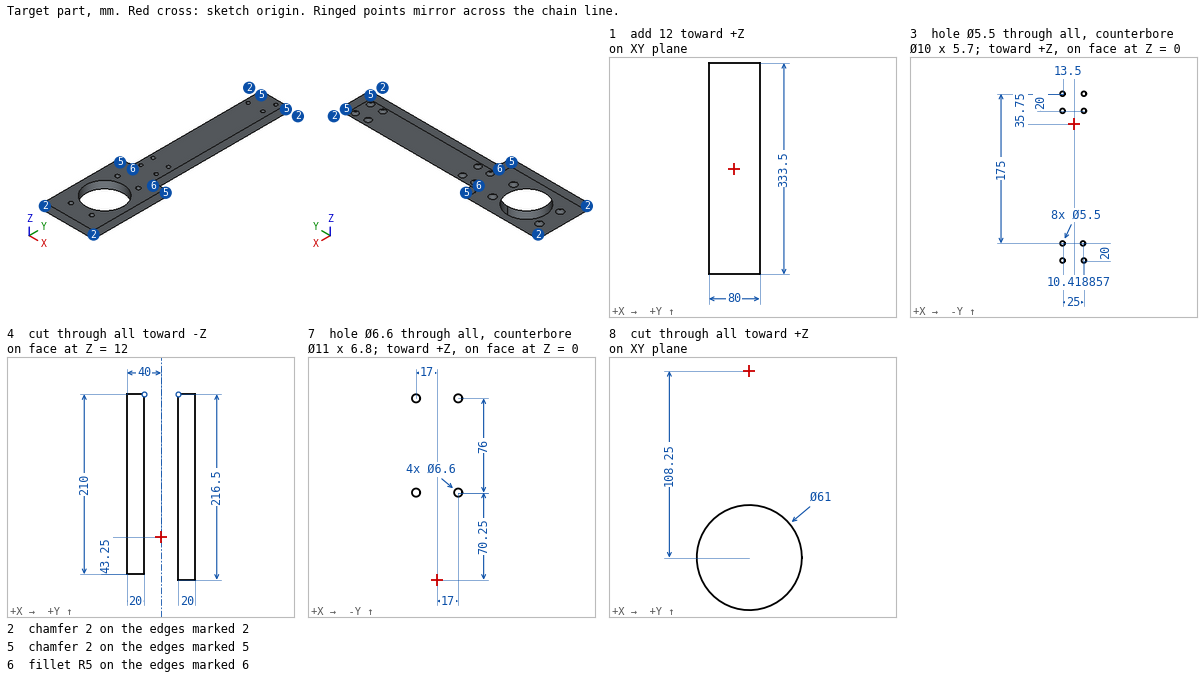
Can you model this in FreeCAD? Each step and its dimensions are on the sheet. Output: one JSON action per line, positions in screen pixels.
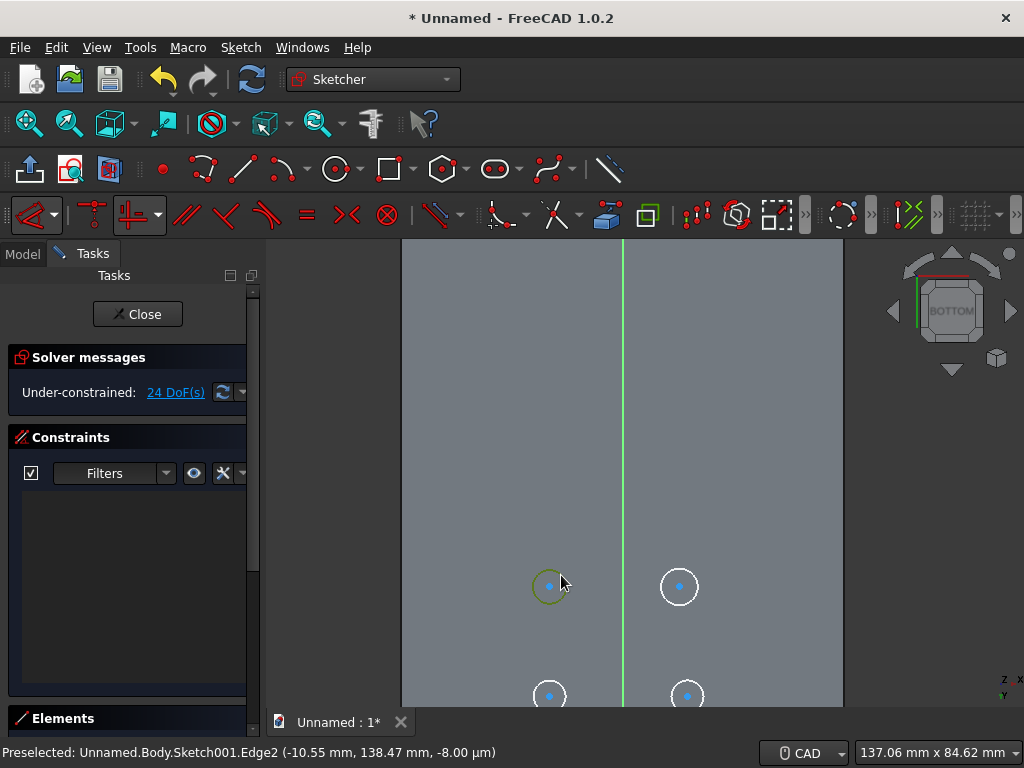
{"action": "scroll", "coordinate": [563, 577], "scroll_direction": "down", "scroll_amount": 7}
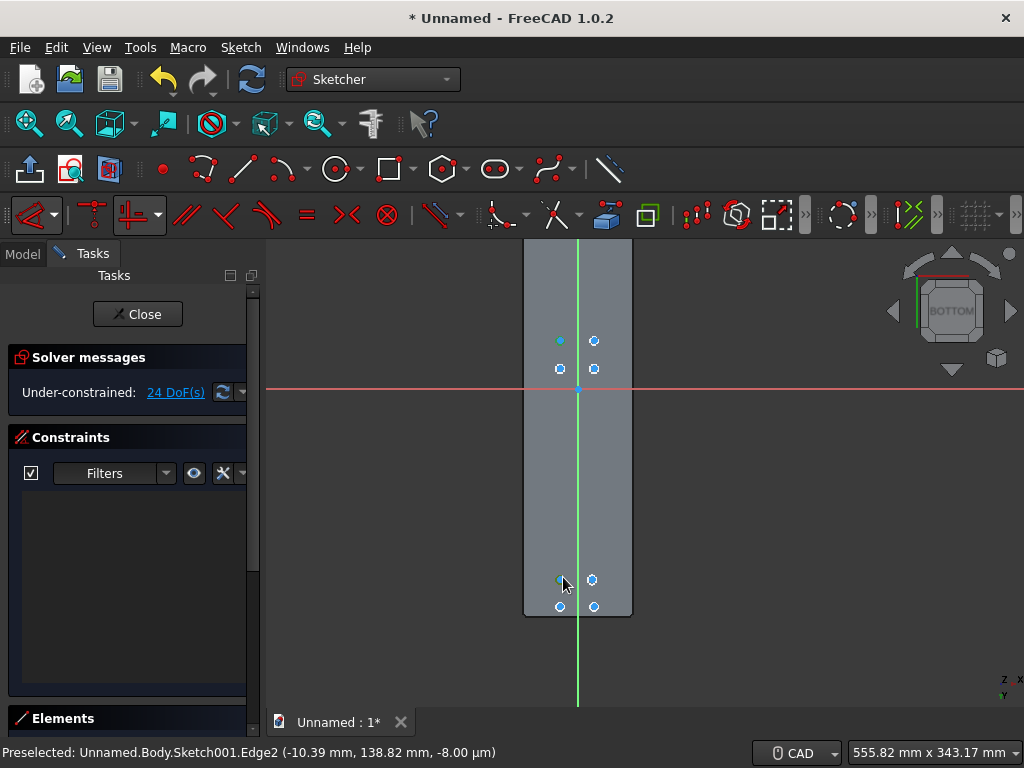
{"action": "scroll", "coordinate": [597, 604], "scroll_direction": "up", "scroll_amount": 7}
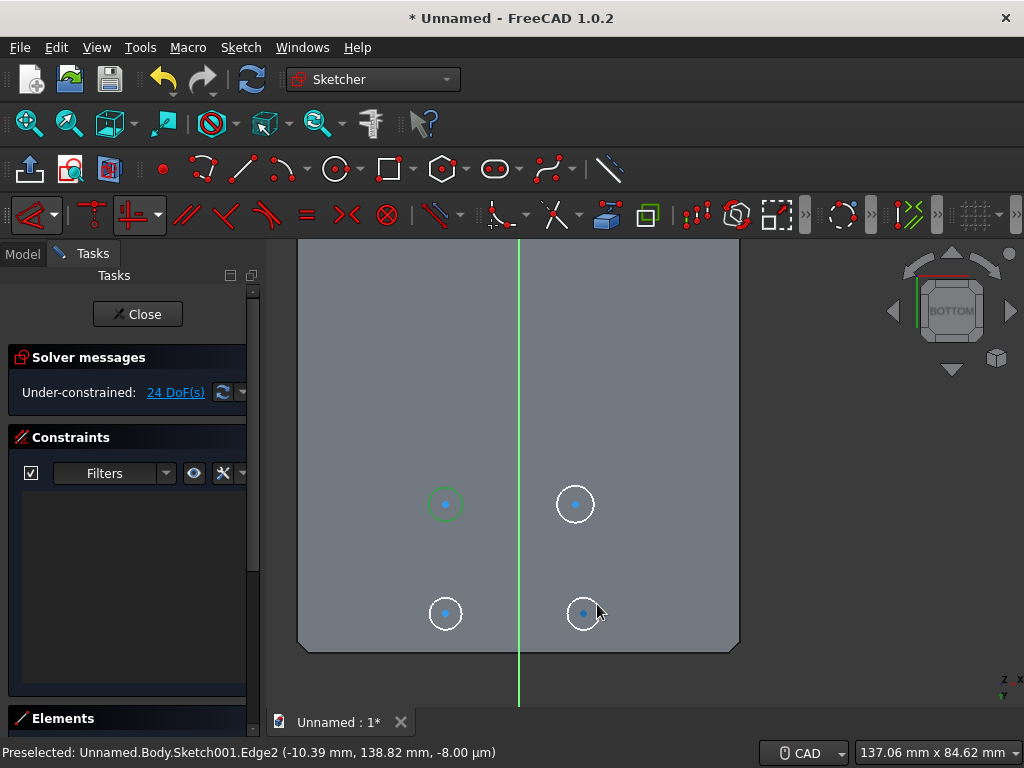
{"action": "left_click", "coordinate": [595, 602]}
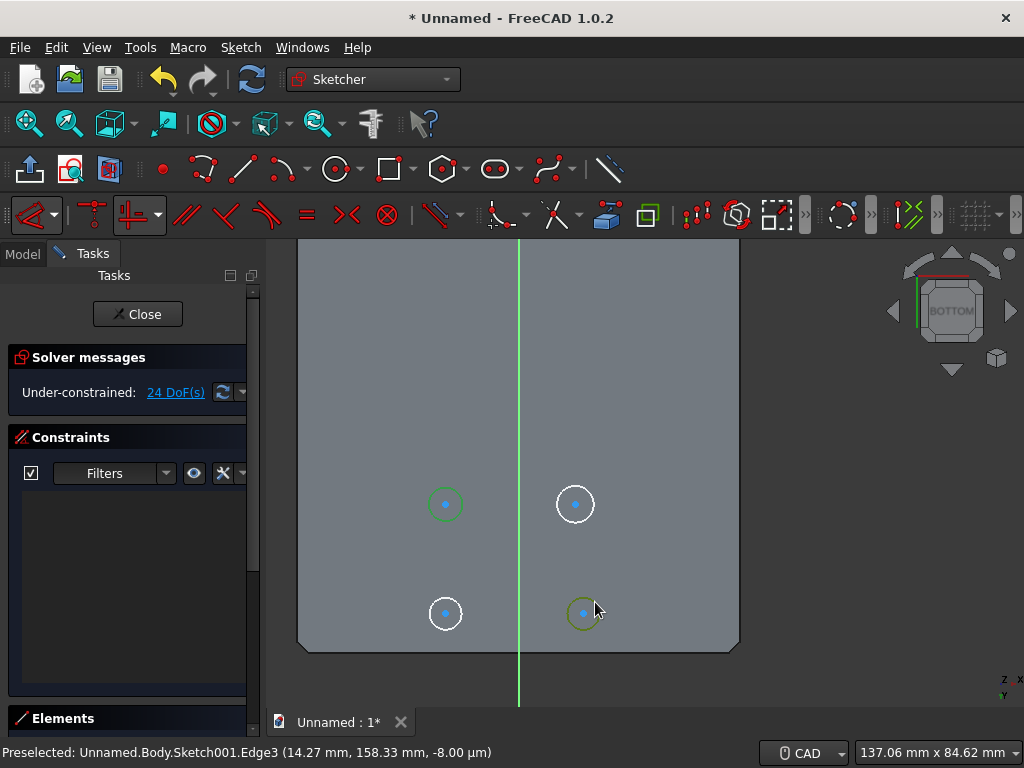
{"action": "left_click", "coordinate": [588, 491]}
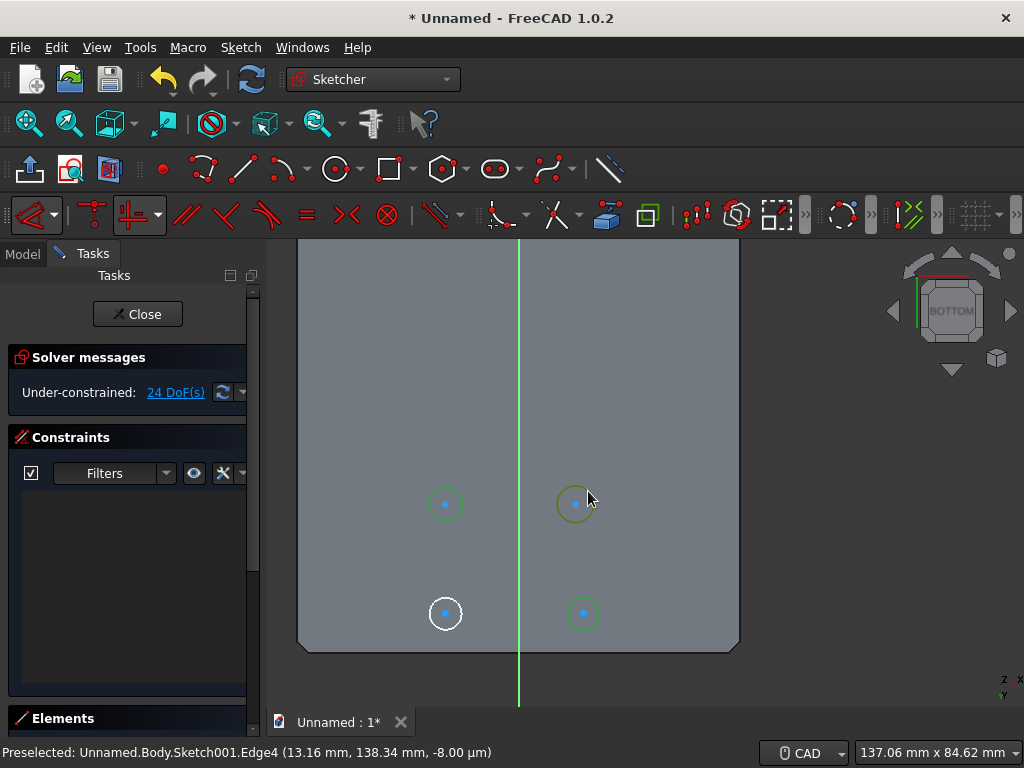
{"action": "left_click", "coordinate": [457, 602]}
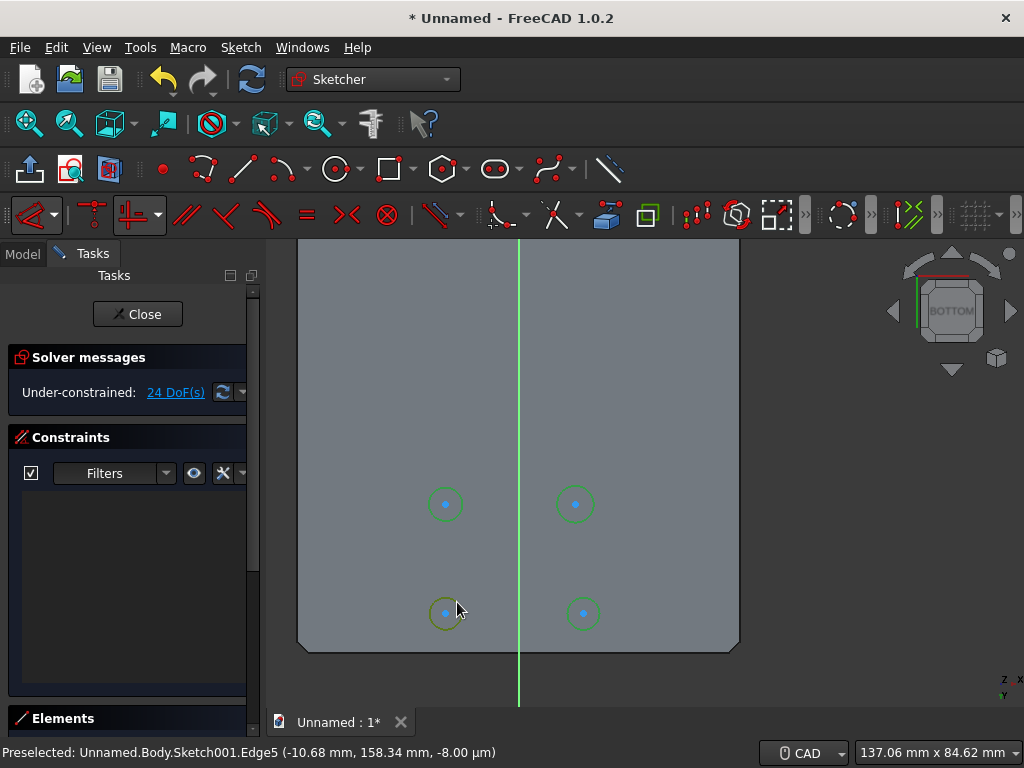
{"action": "scroll", "coordinate": [597, 604], "scroll_direction": "down", "scroll_amount": 7}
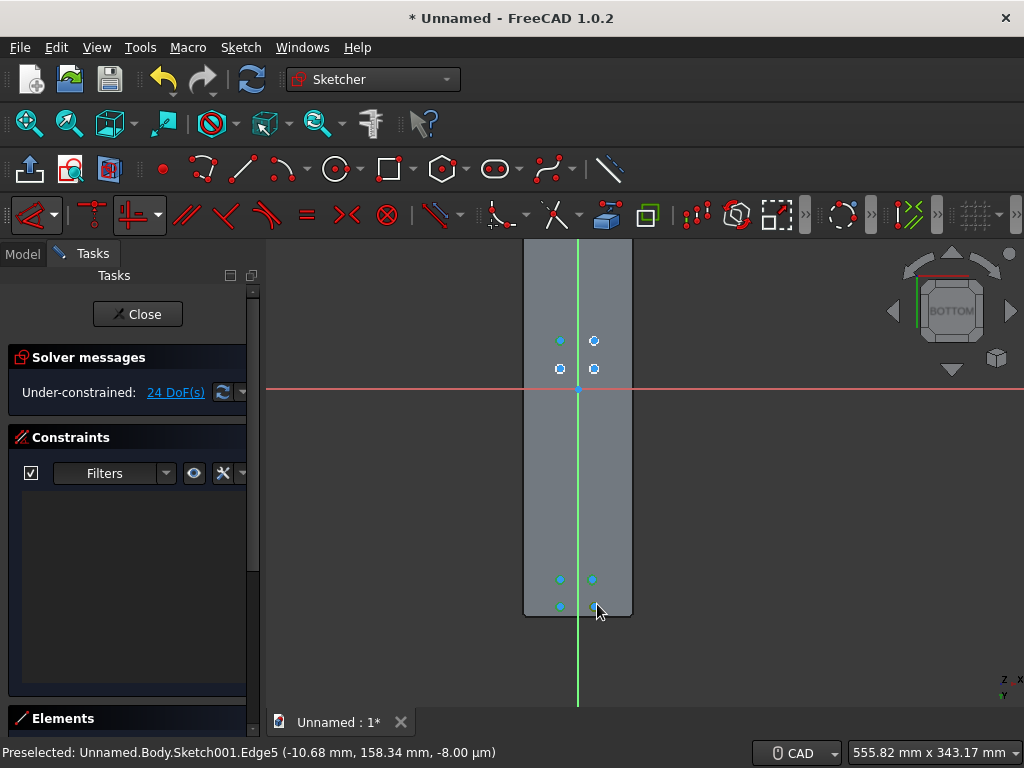
{"action": "scroll", "coordinate": [597, 366], "scroll_direction": "up", "scroll_amount": 6}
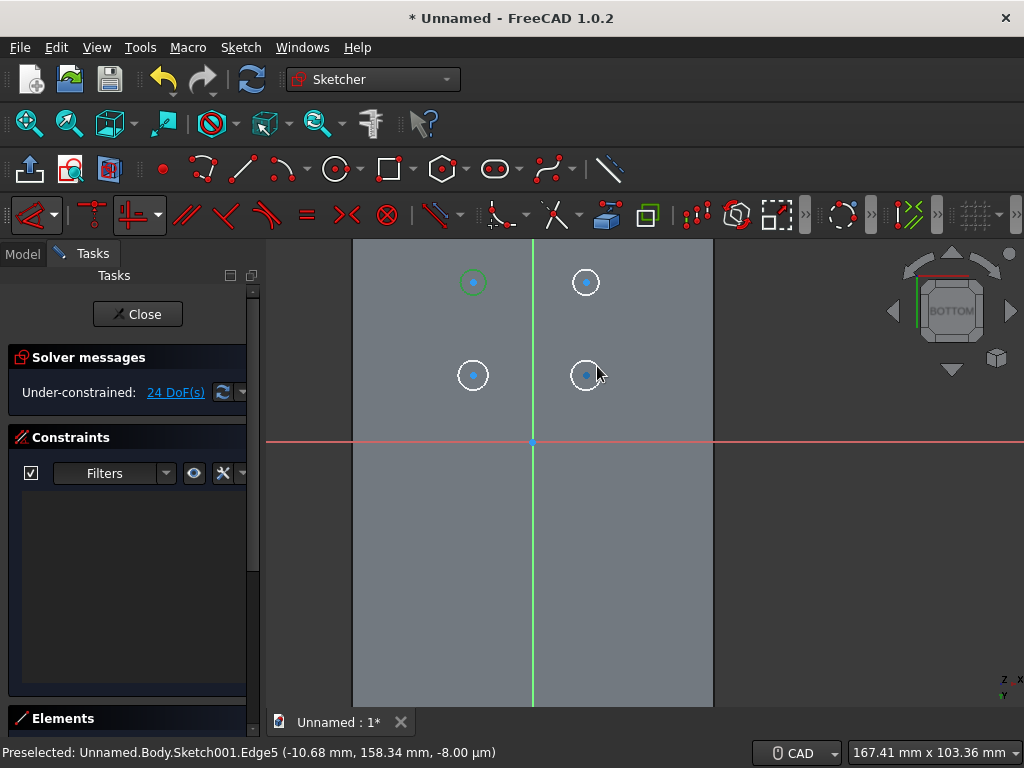
{"action": "left_click", "coordinate": [596, 365]}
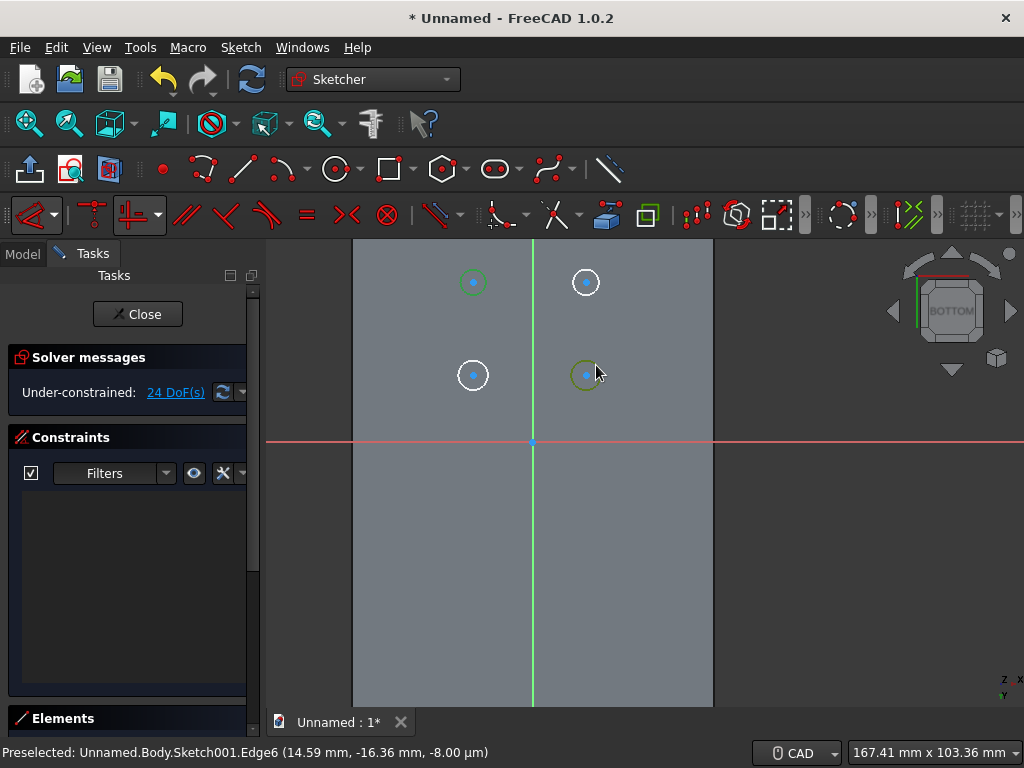
{"action": "left_click", "coordinate": [484, 365]}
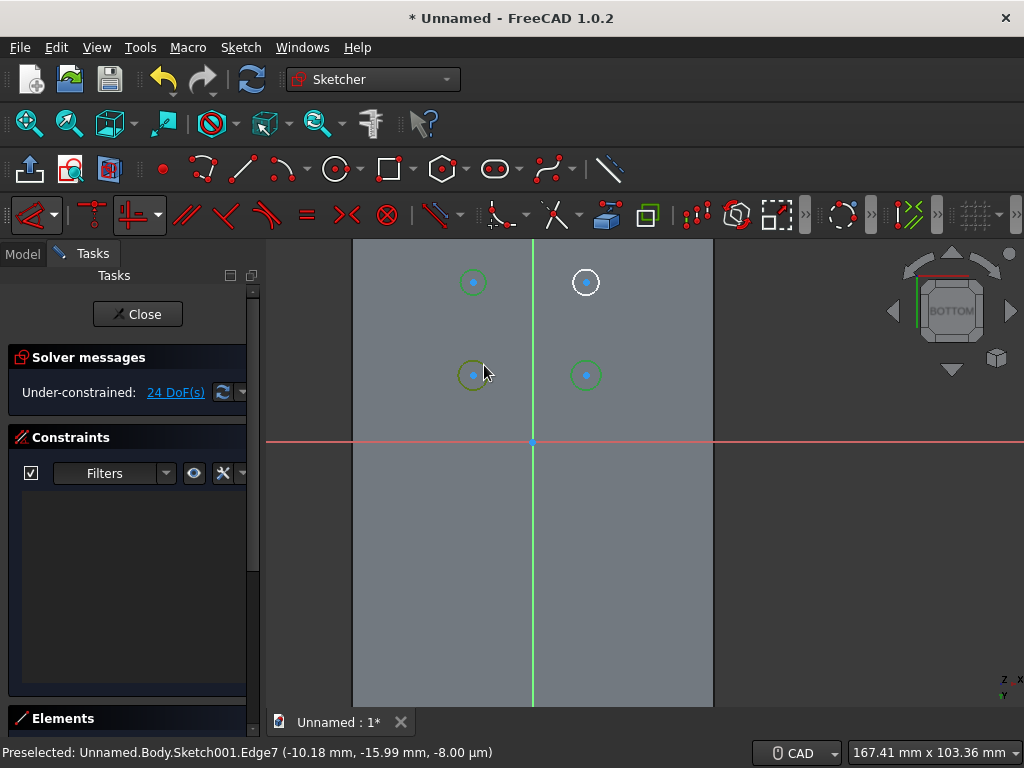
{"action": "left_click", "coordinate": [595, 273]}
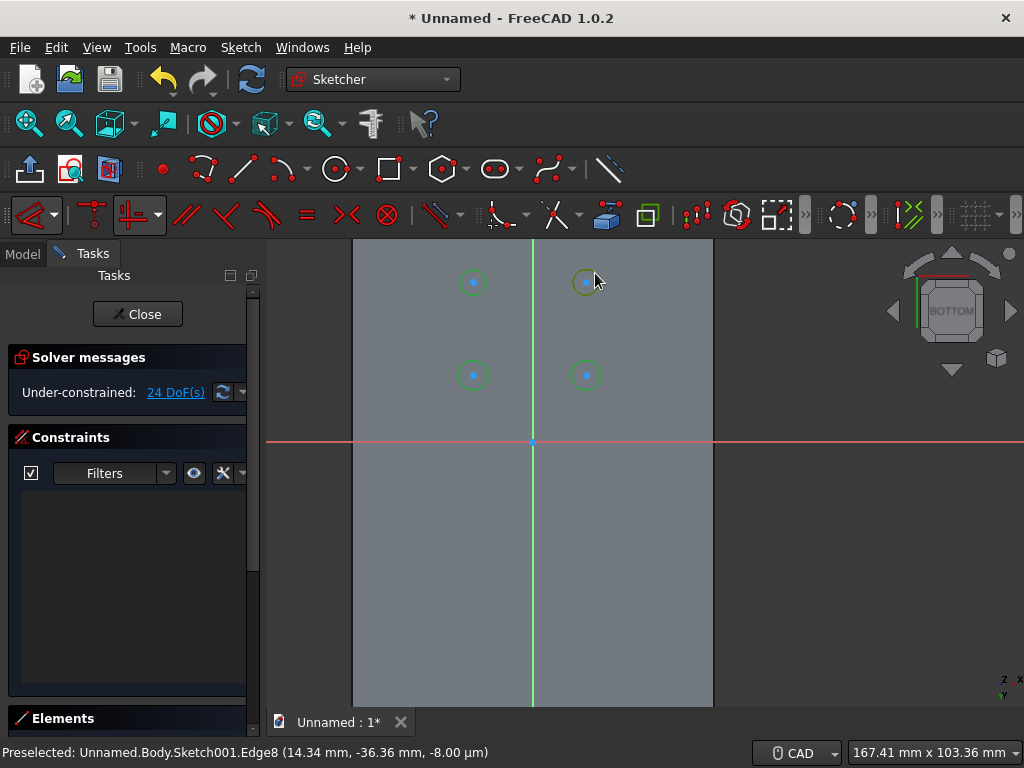
{"action": "key", "text": "e"}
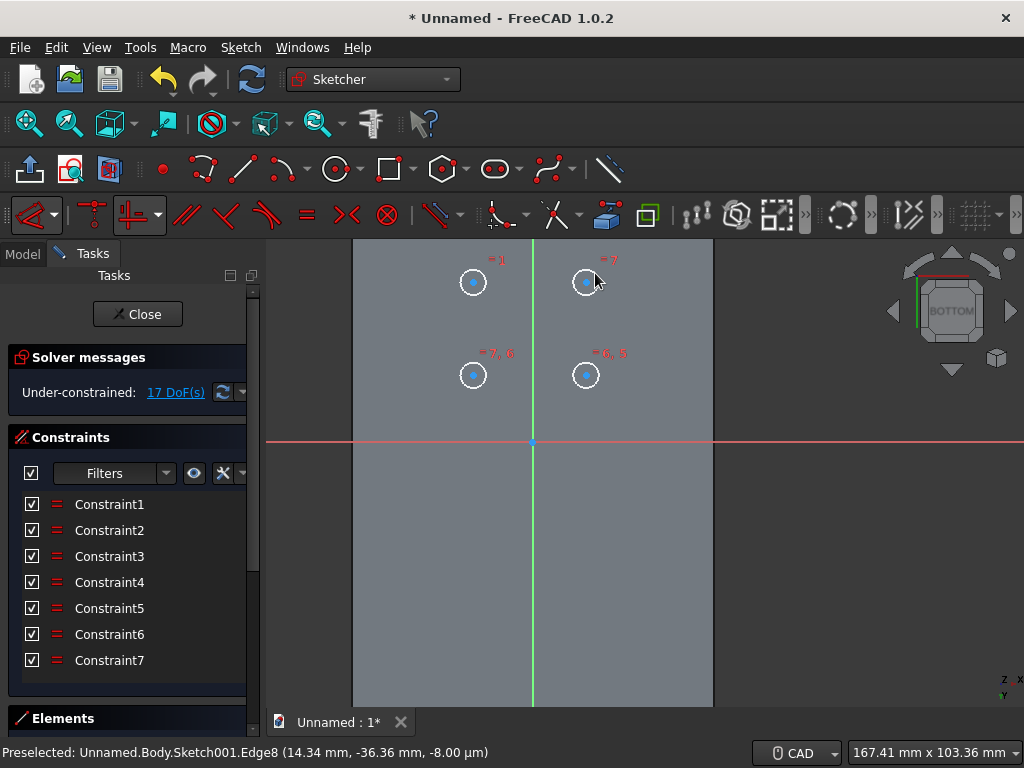
{"action": "scroll", "coordinate": [597, 366], "scroll_direction": "down", "scroll_amount": 6}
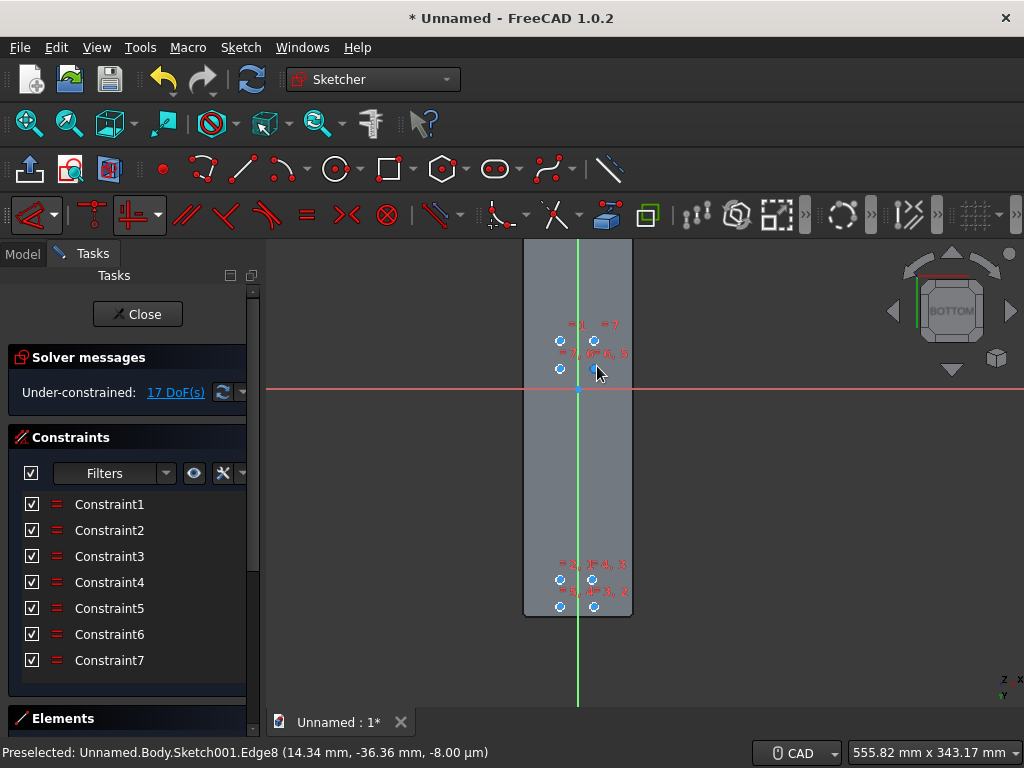
{"action": "left_click", "coordinate": [560, 341]}